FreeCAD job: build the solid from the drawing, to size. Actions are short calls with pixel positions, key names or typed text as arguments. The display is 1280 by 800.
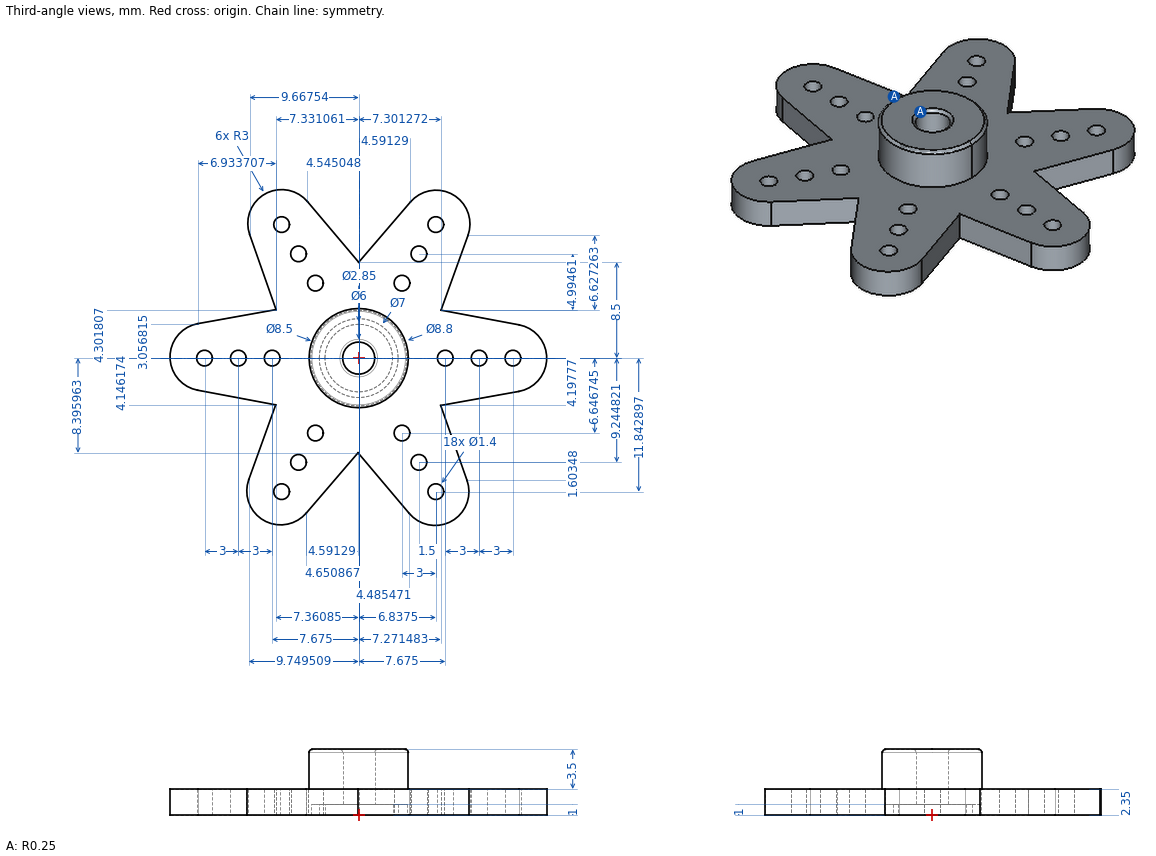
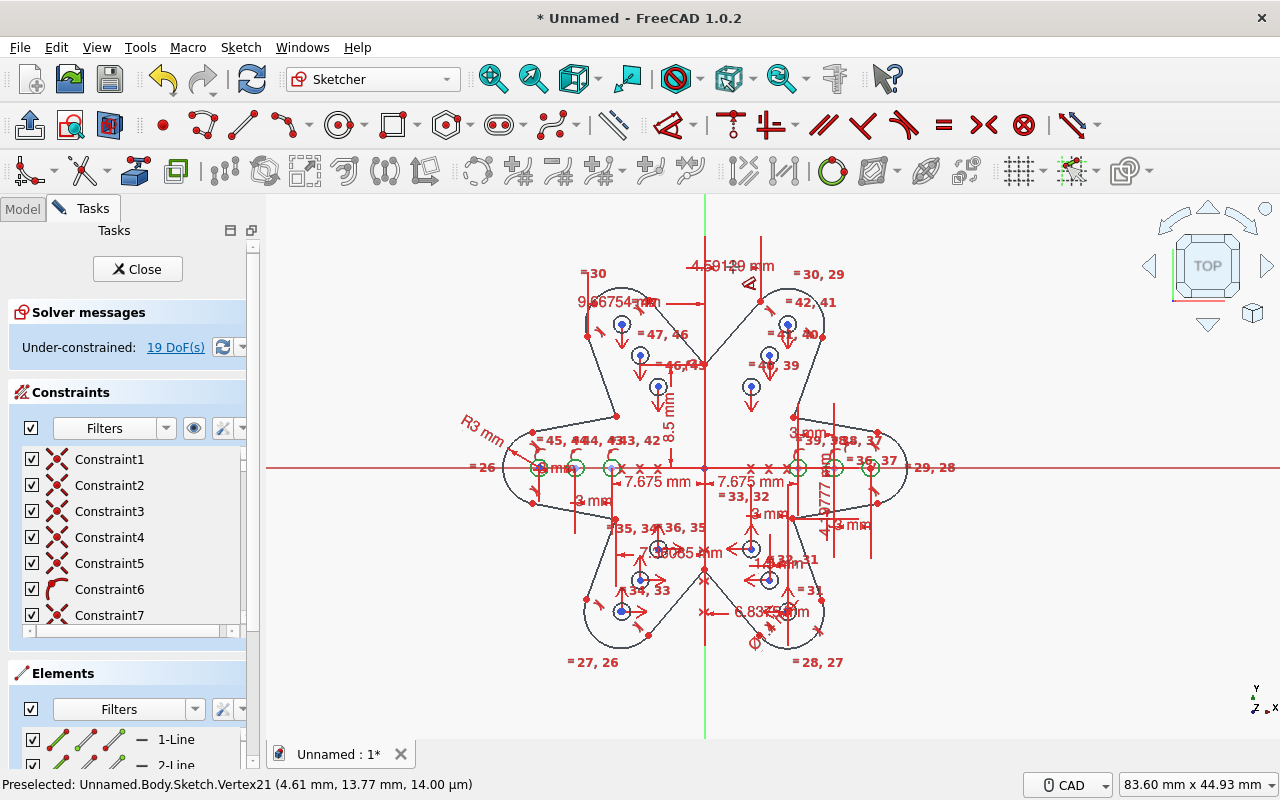
click(665, 616)
click(676, 670)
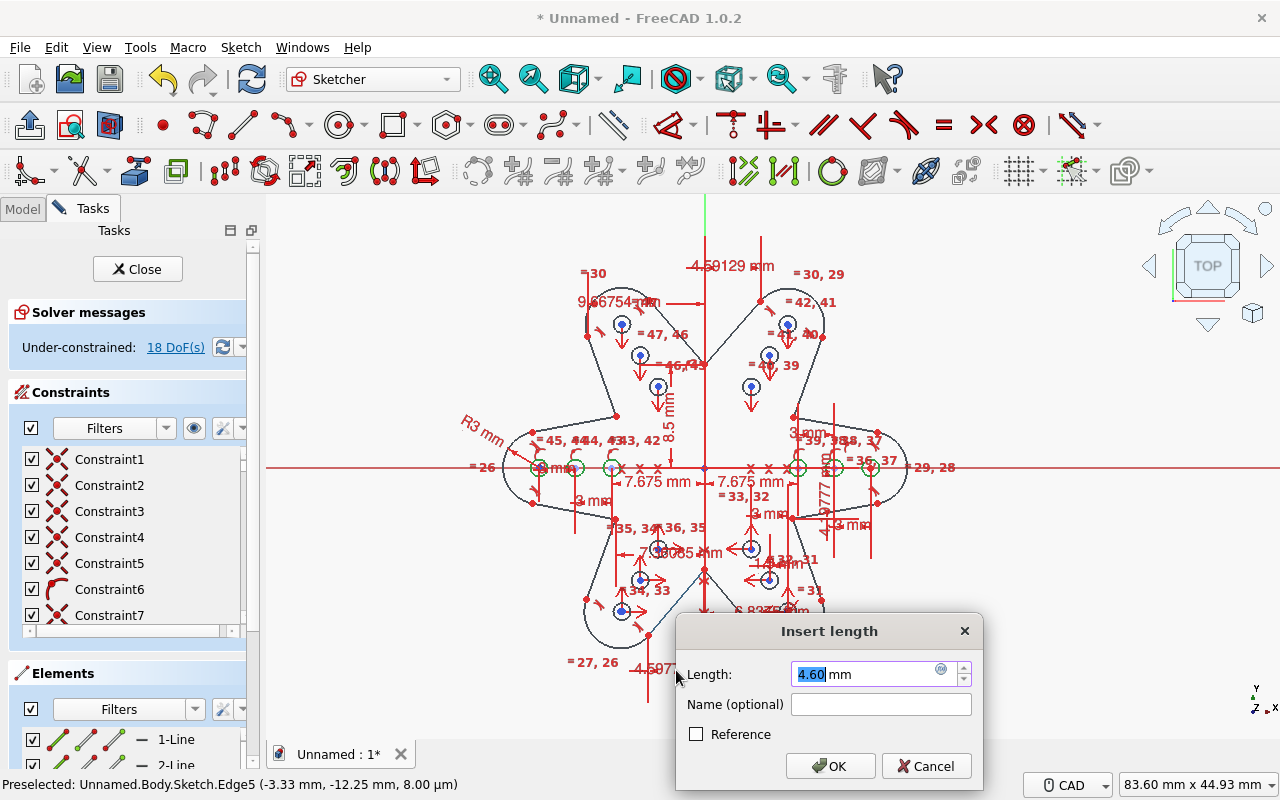
text(4.59129)
key(Return)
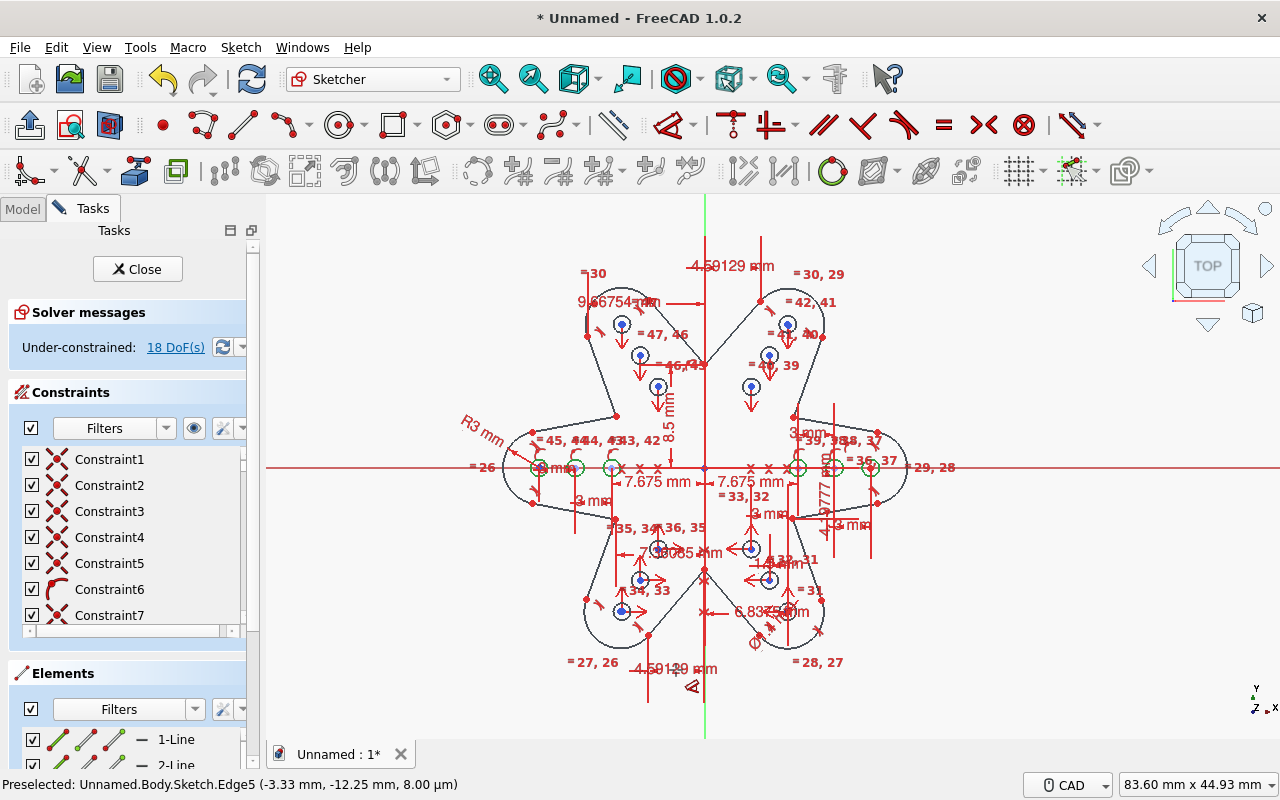
click(770, 580)
click(671, 524)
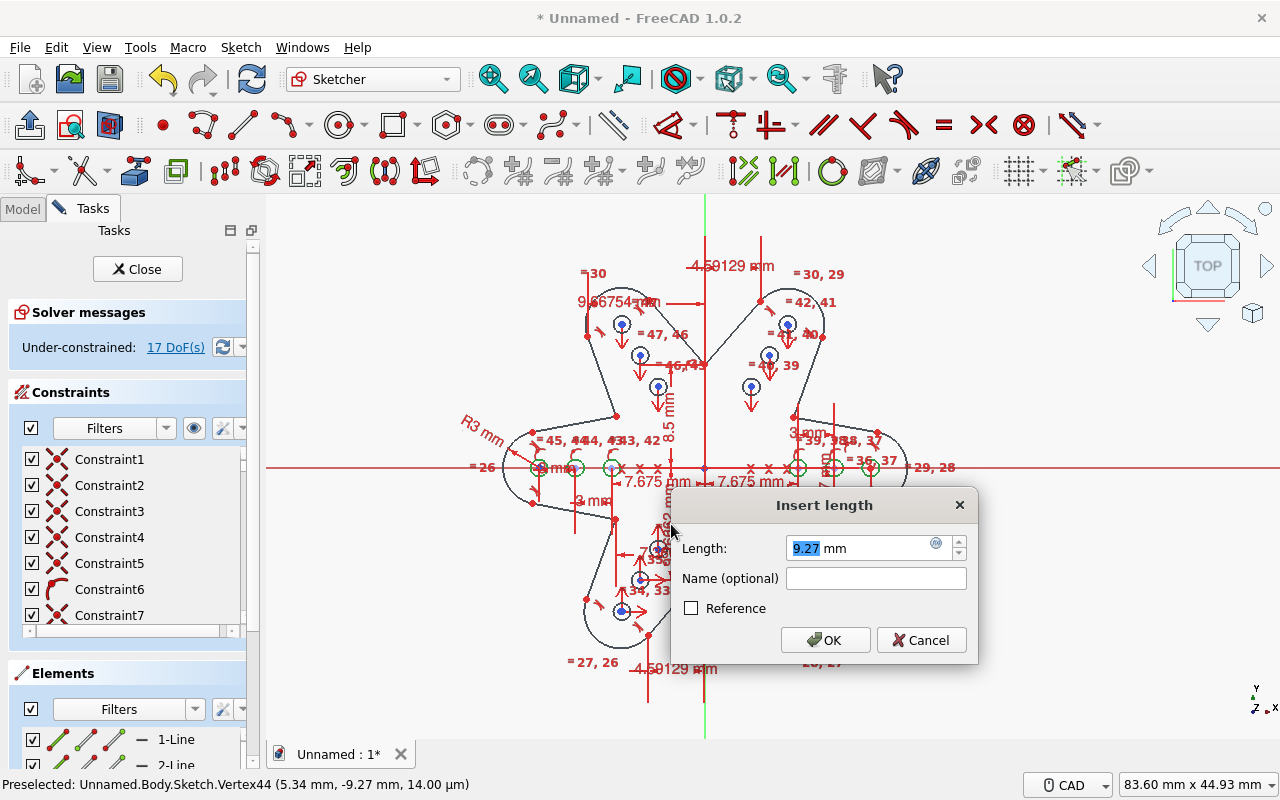
text(9.244821)
key(Return)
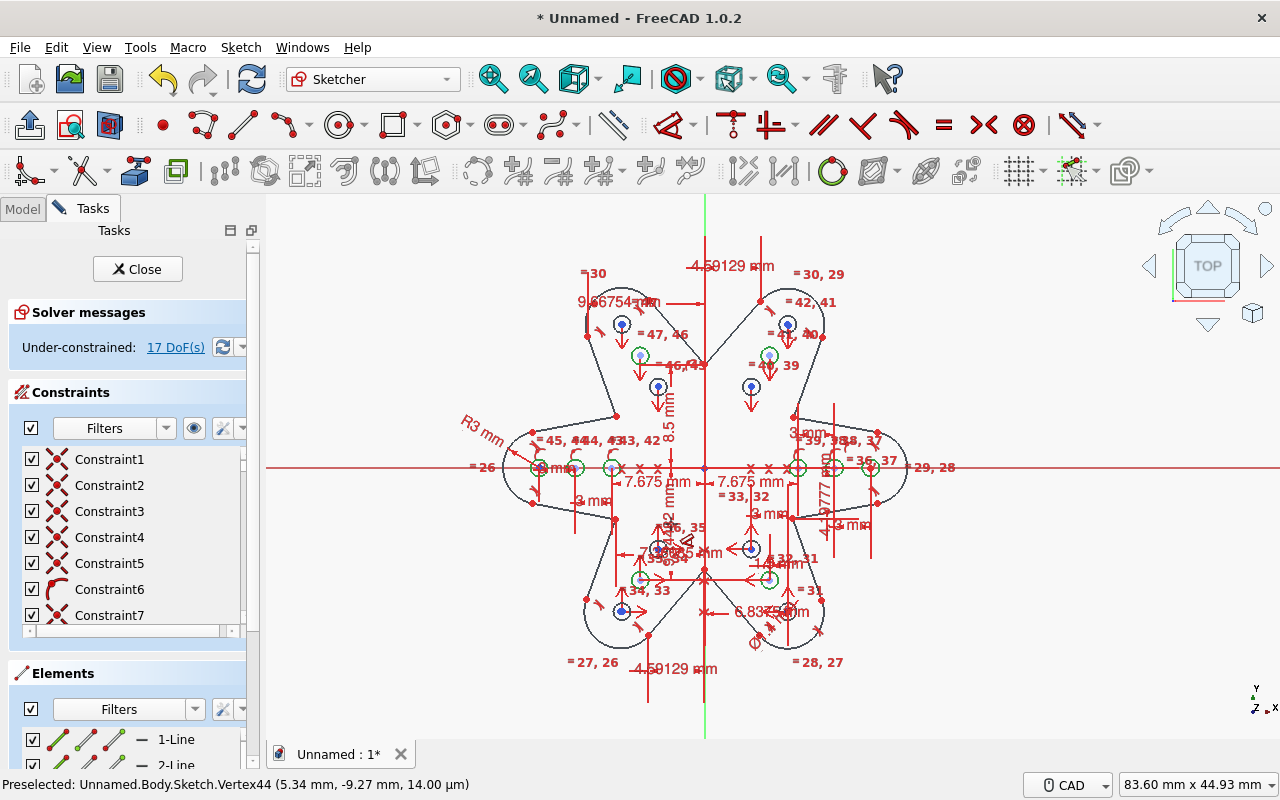
click(751, 549)
click(575, 527)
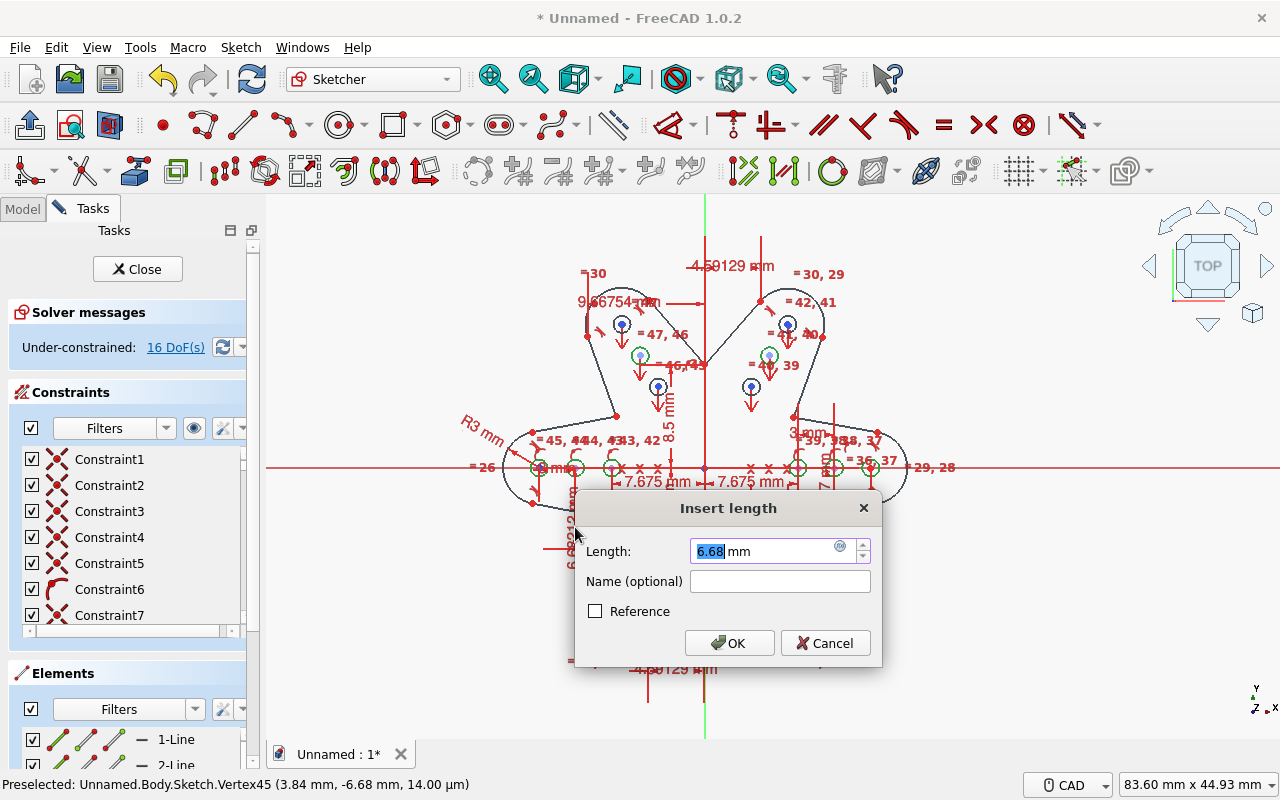
text(6.646745)
key(Return)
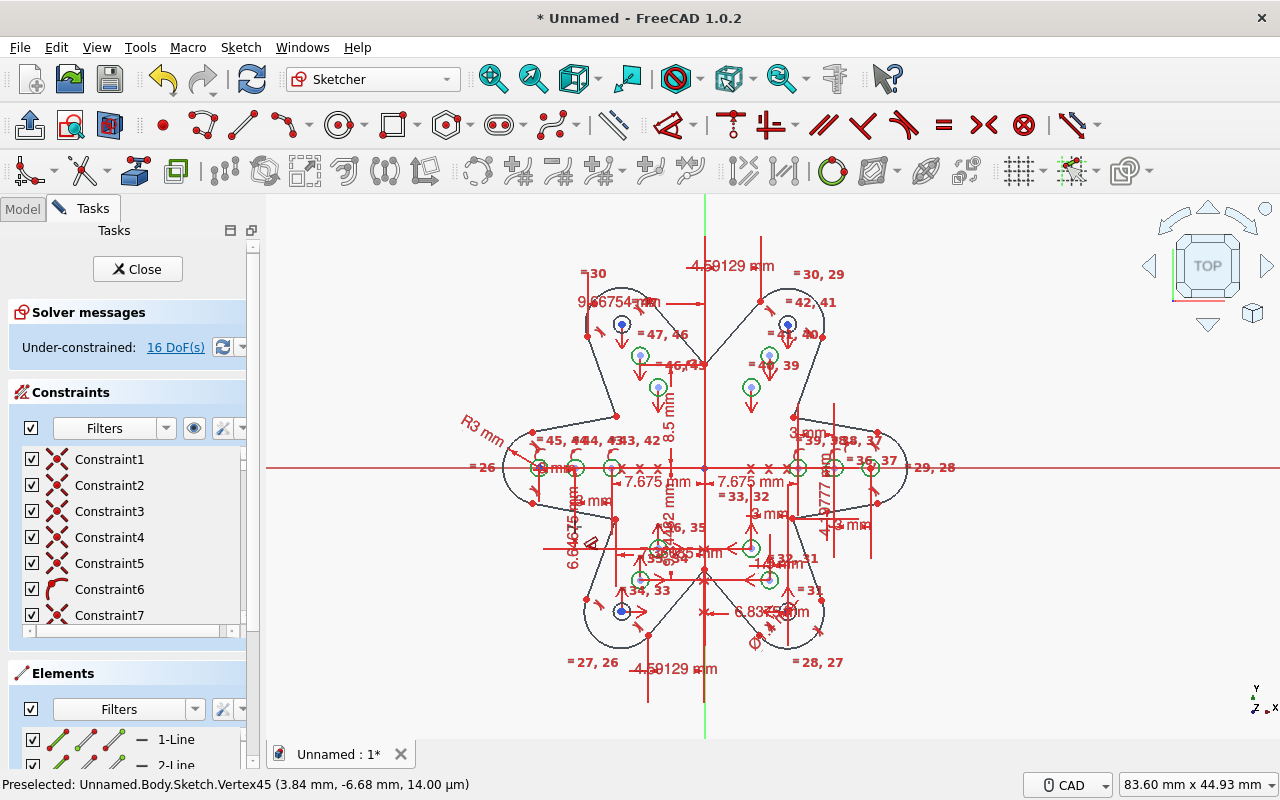
scroll(822, 600, up, 4)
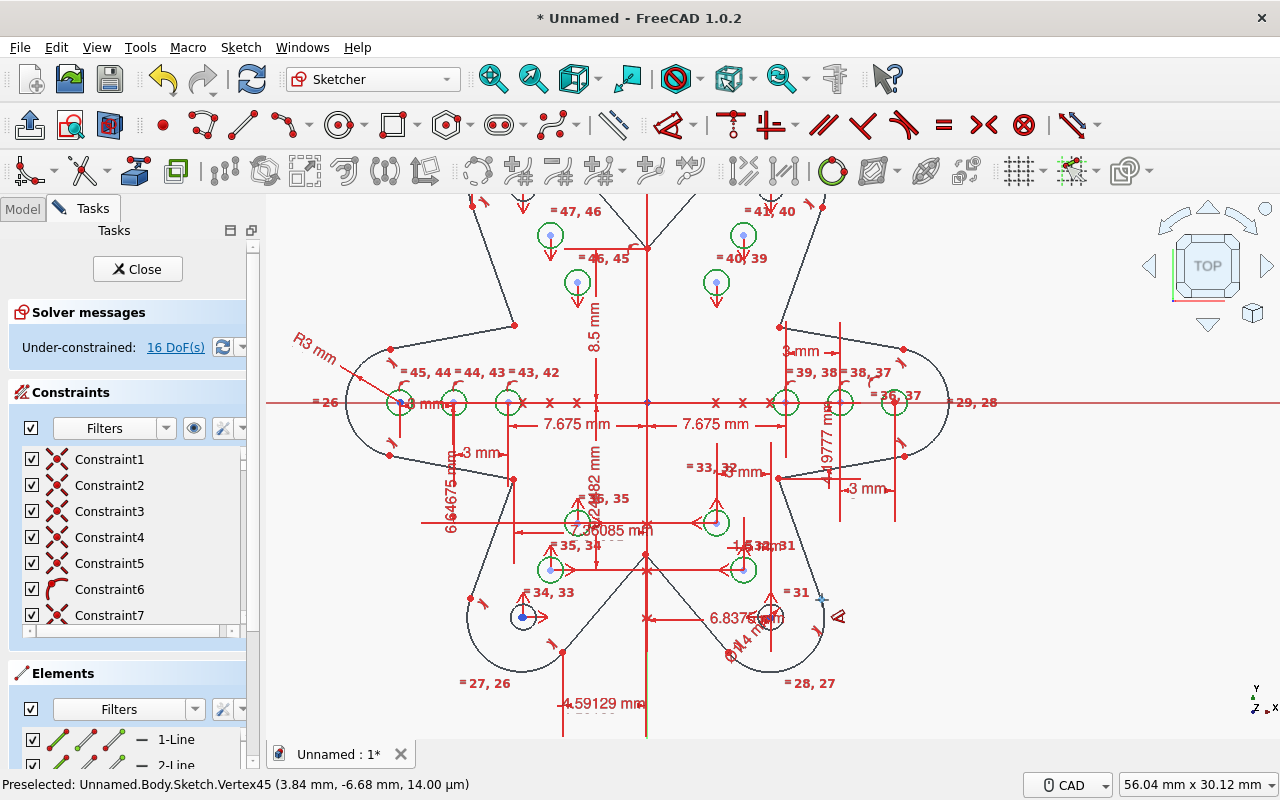
click(821, 599)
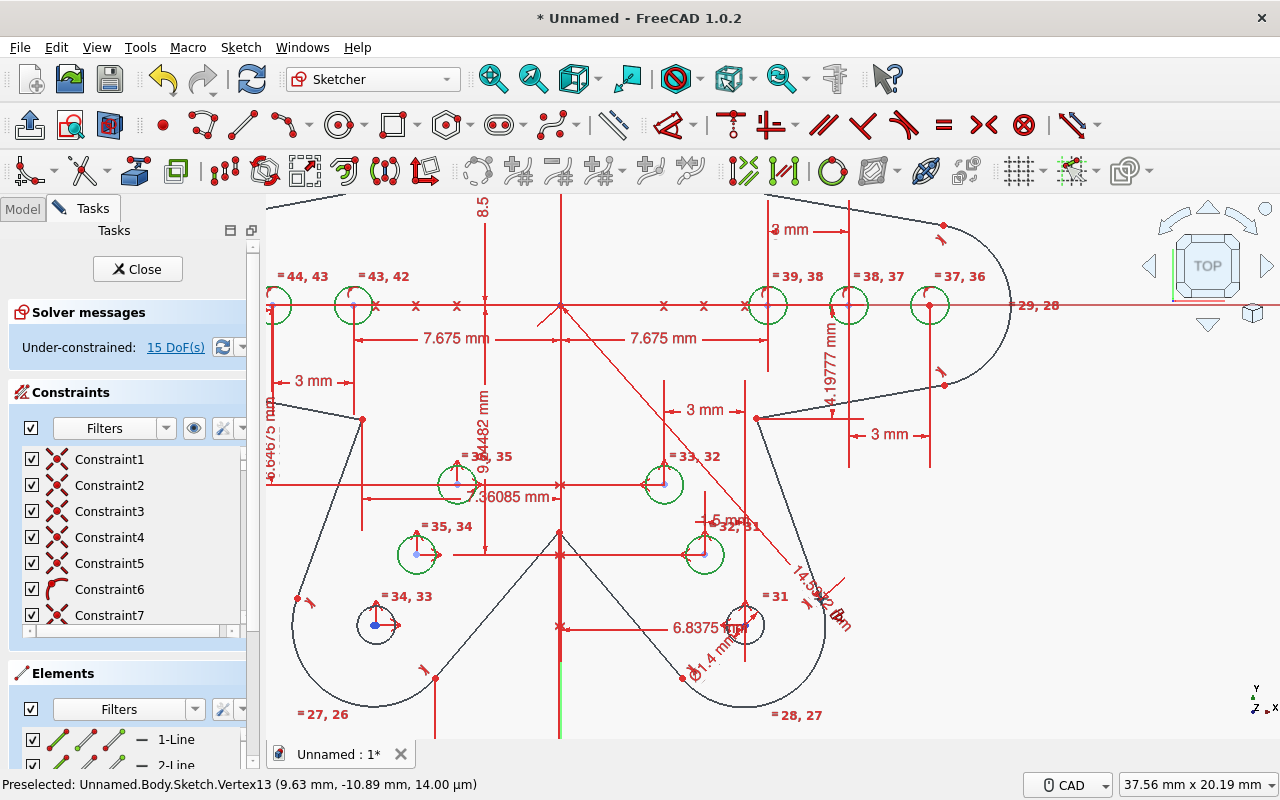
click(705, 555)
click(855, 577)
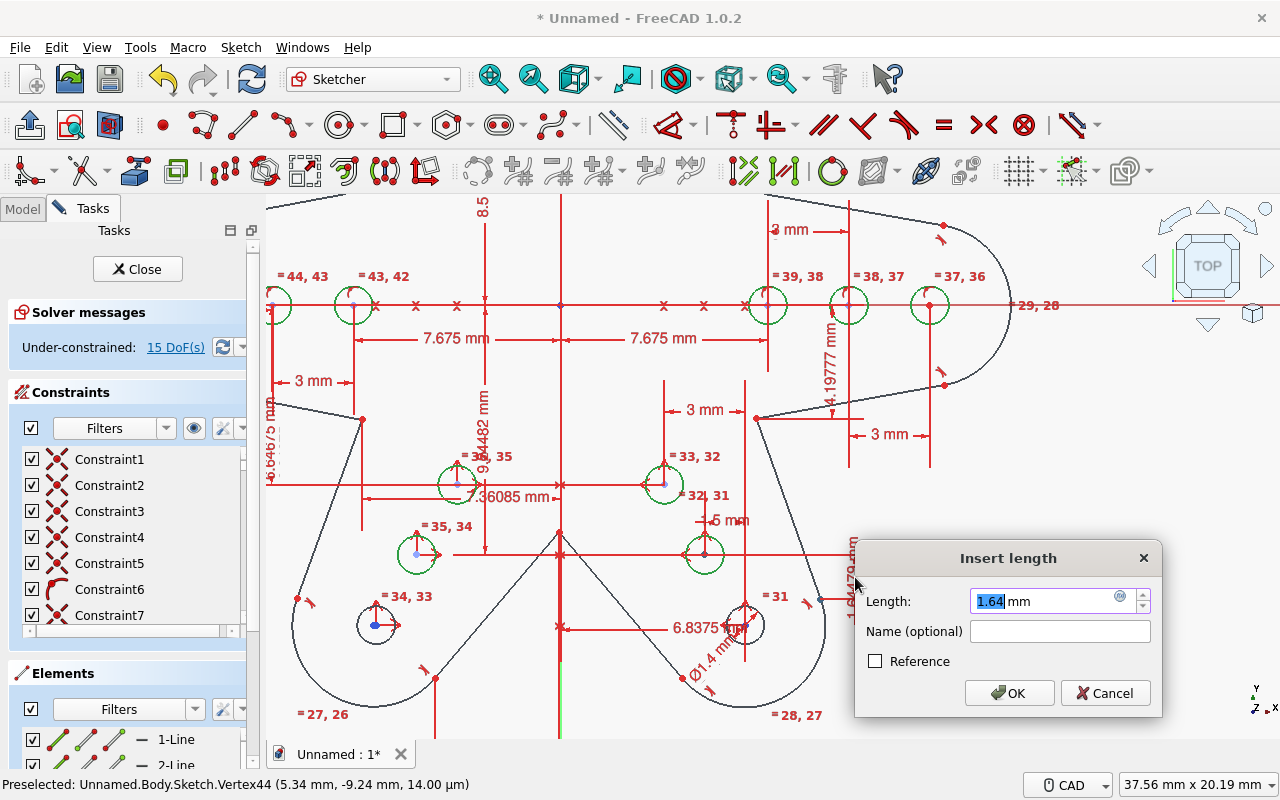
text(1.60348)
key(Return)